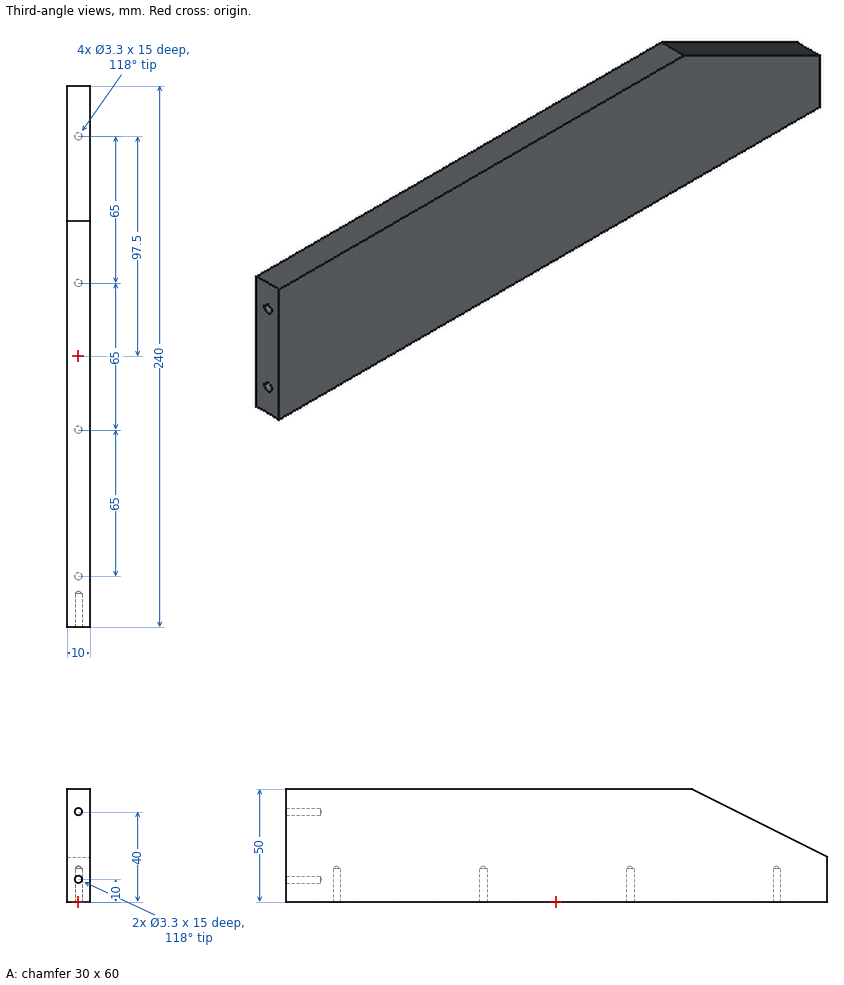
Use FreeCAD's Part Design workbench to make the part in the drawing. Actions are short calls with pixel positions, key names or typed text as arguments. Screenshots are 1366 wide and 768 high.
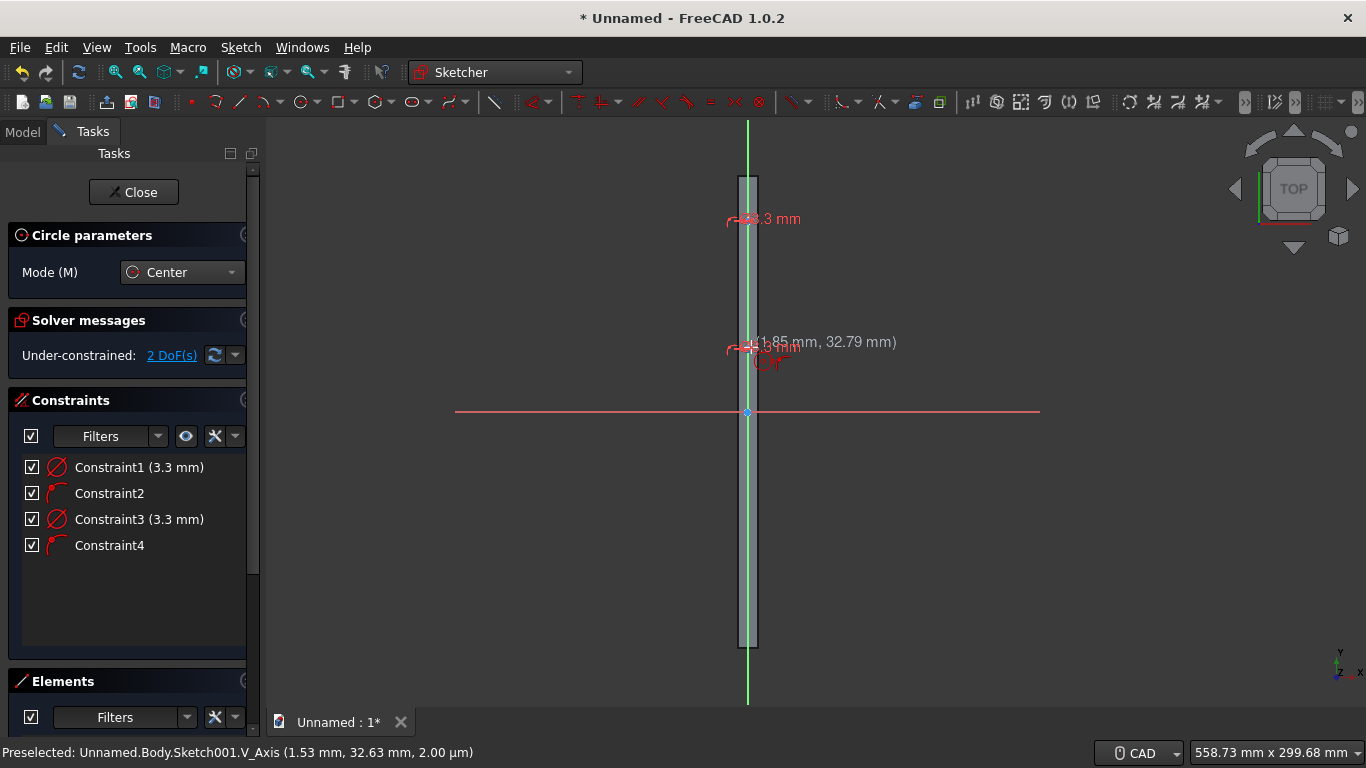
scroll(748, 476, up, 10)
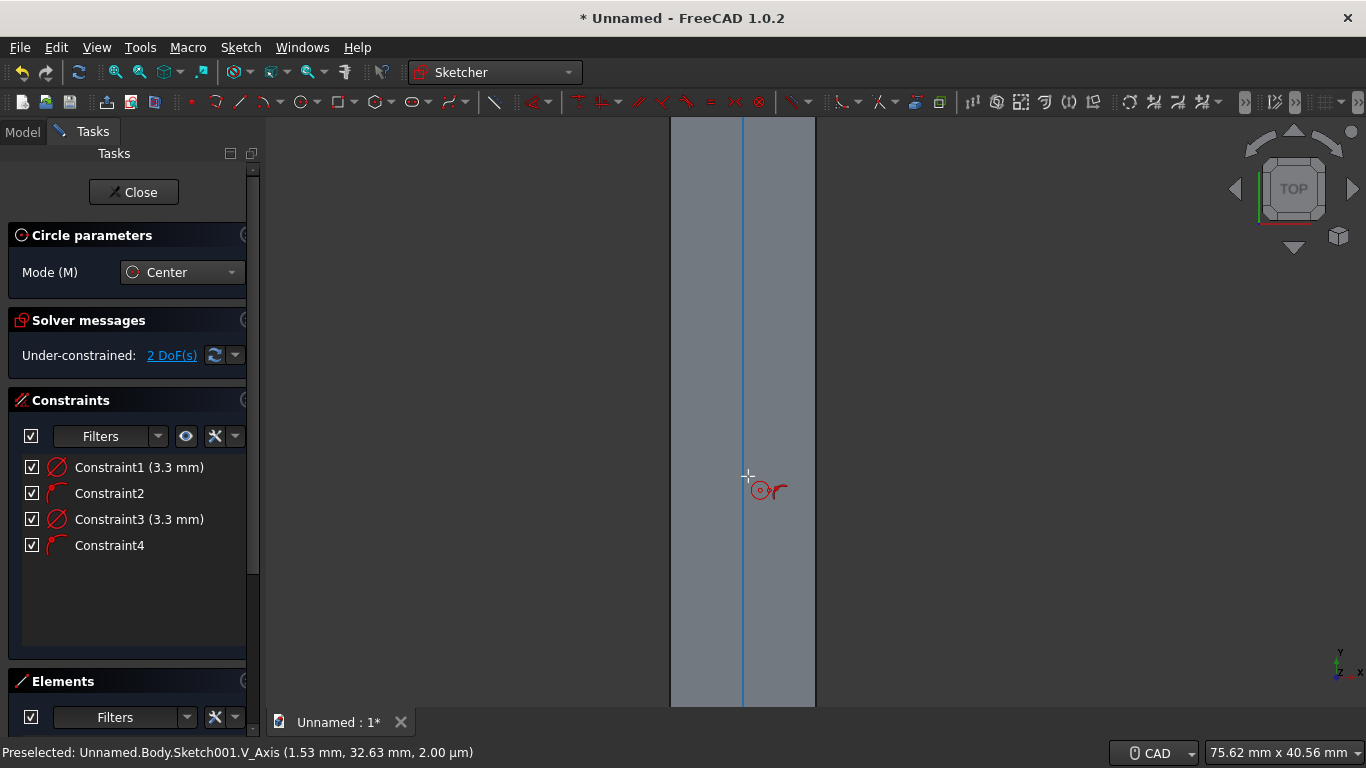
scroll(748, 477, down, 10)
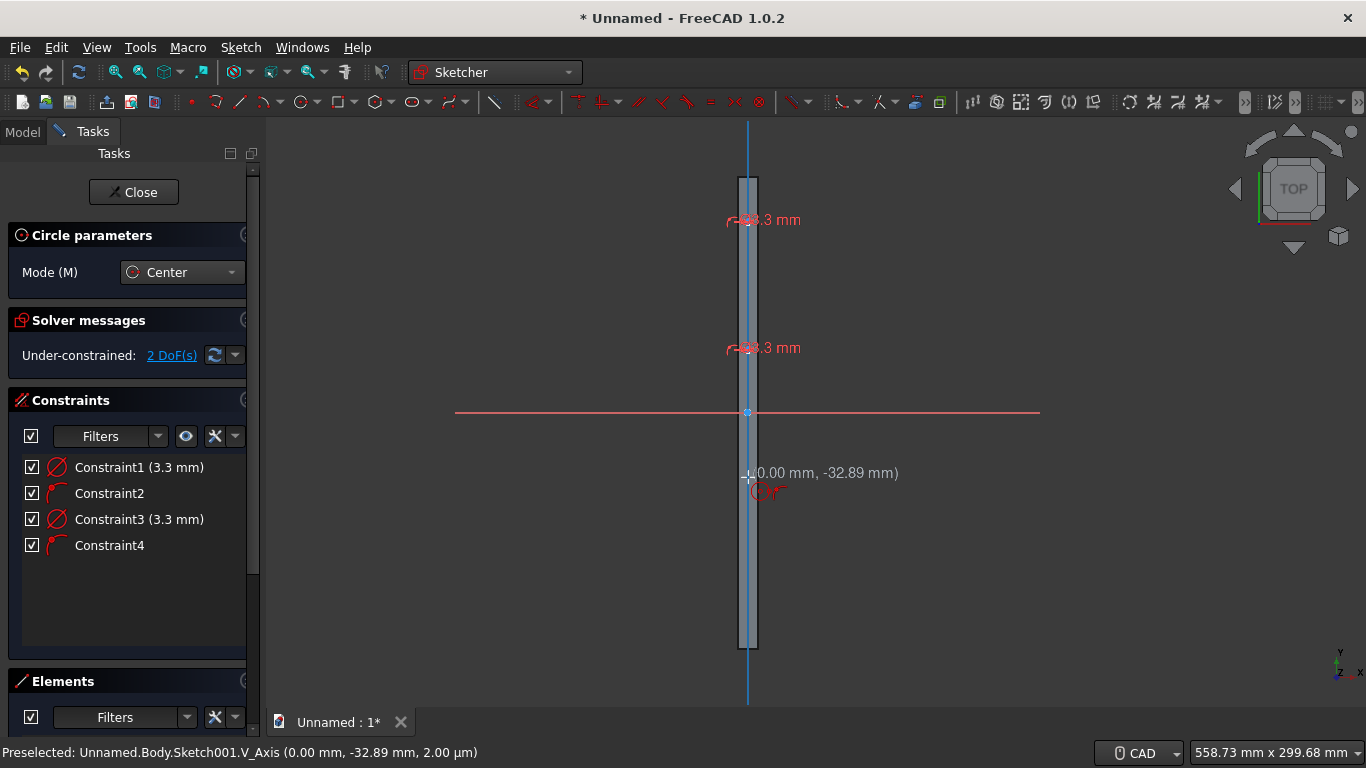
click(748, 477)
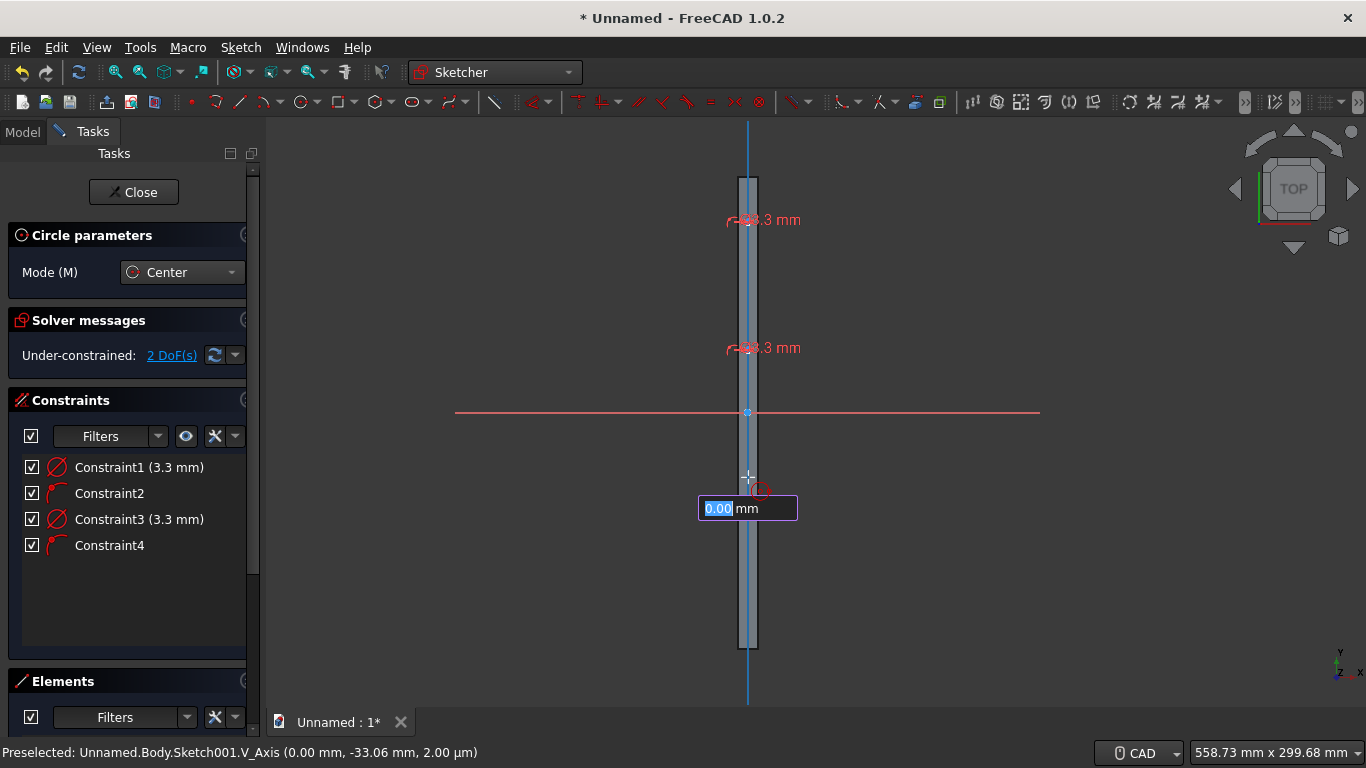
scroll(751, 476, up, 9)
move(747, 472)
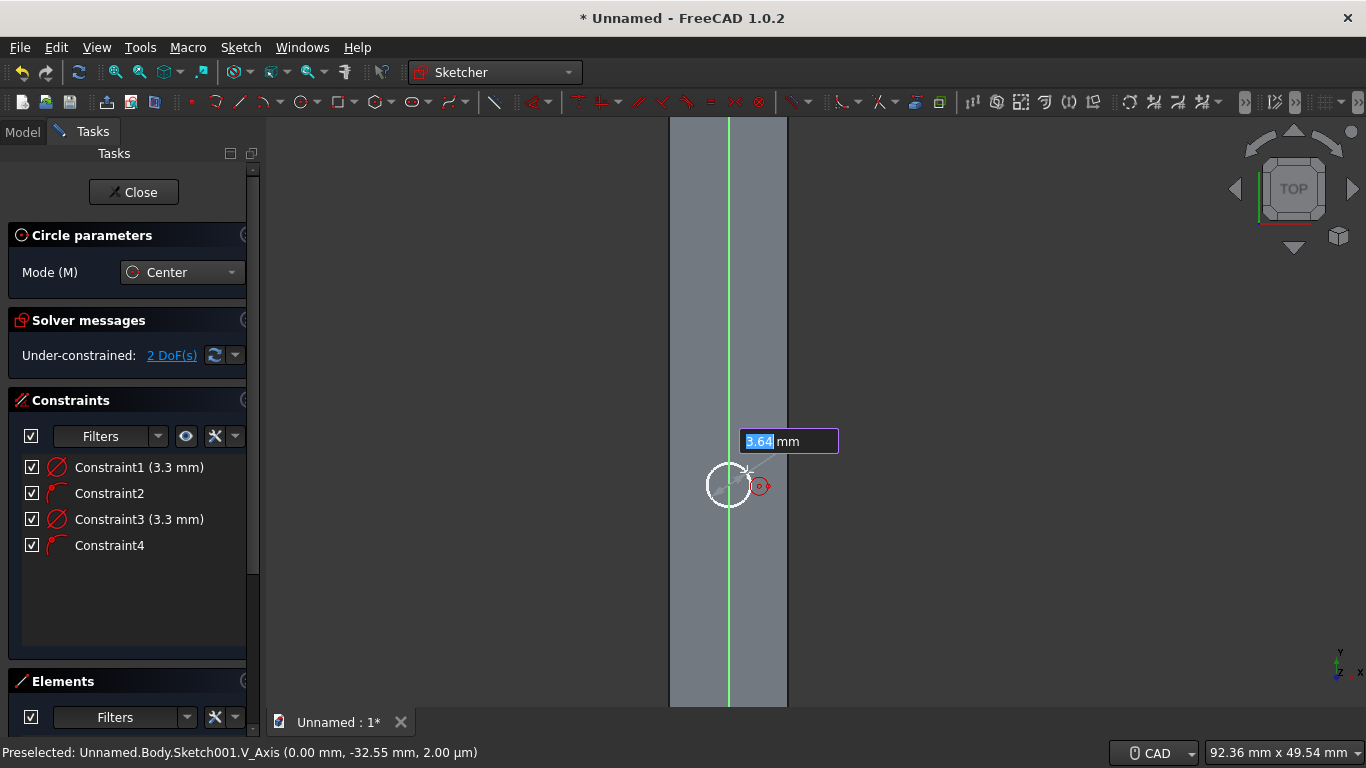
text(3.3)
key(Return)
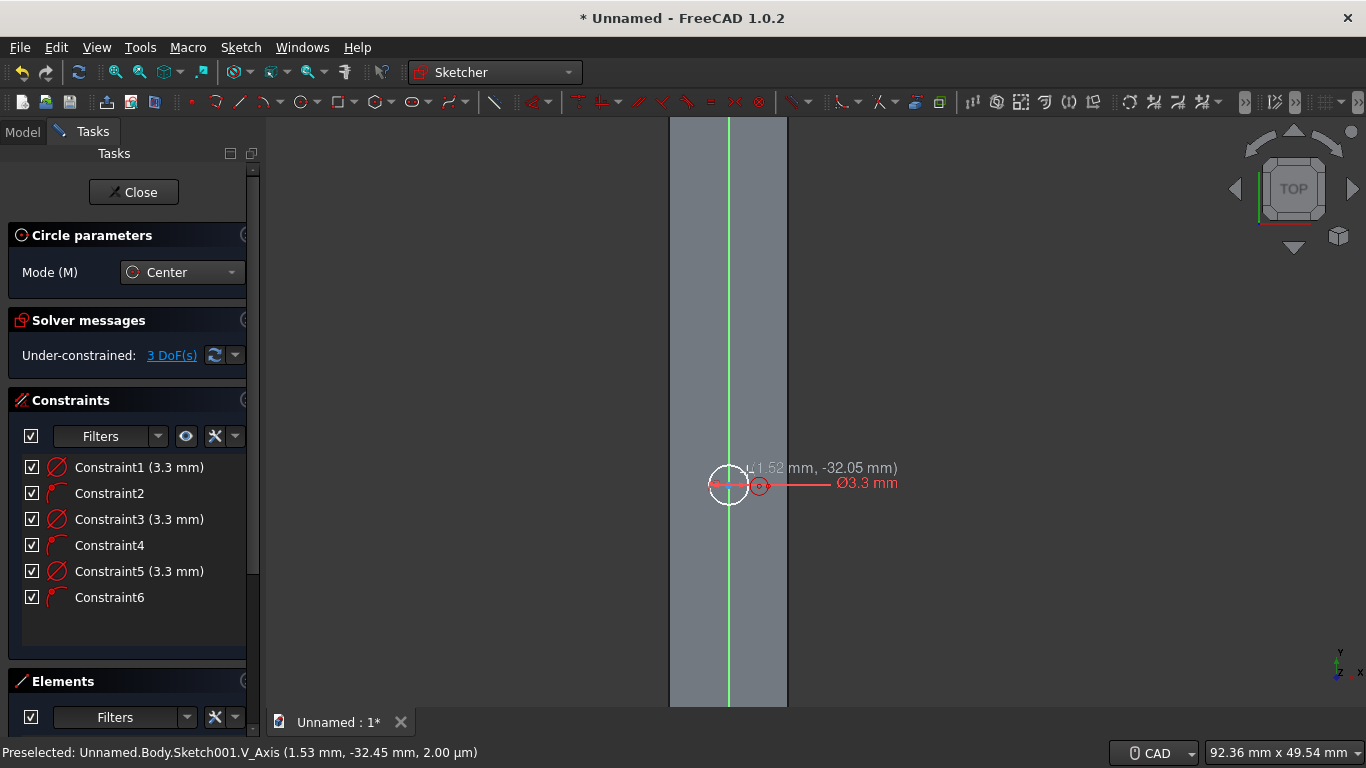
scroll(751, 476, down, 9)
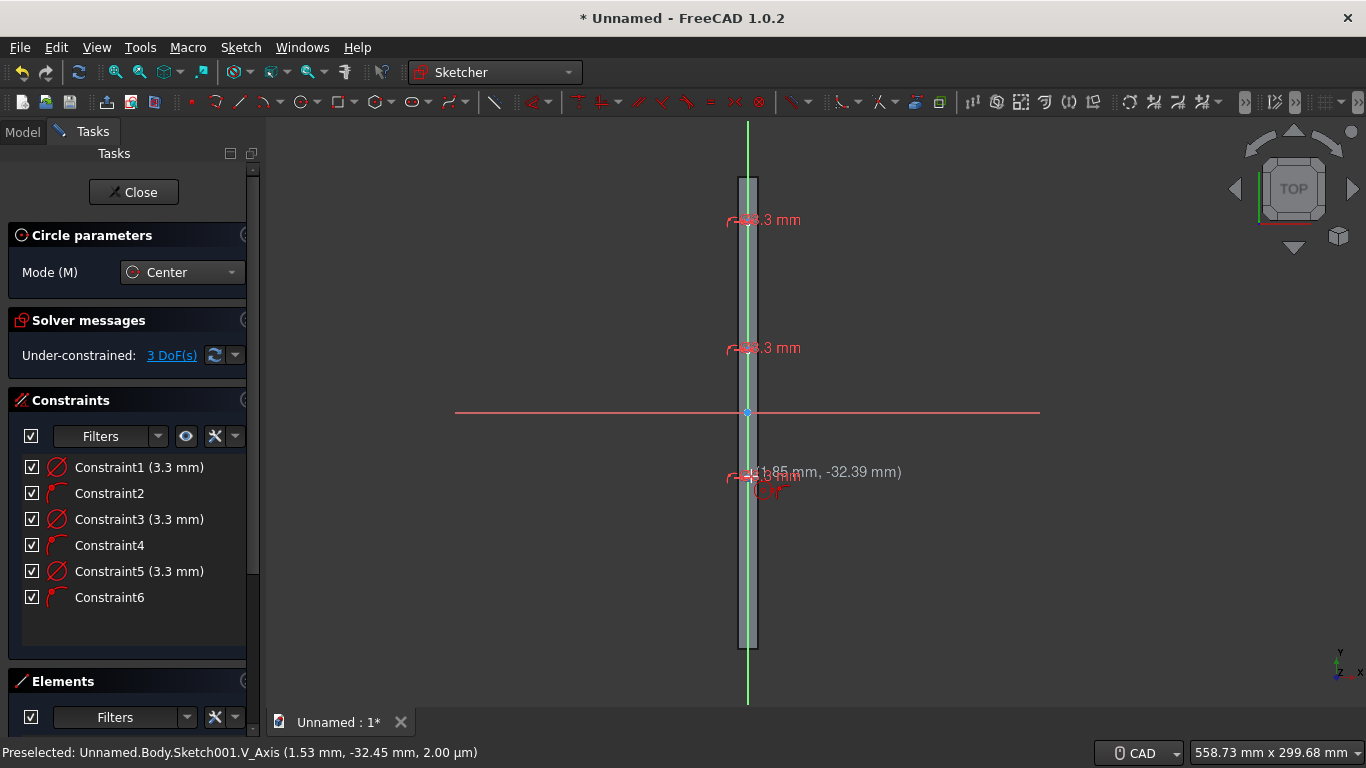
scroll(748, 605, up, 10)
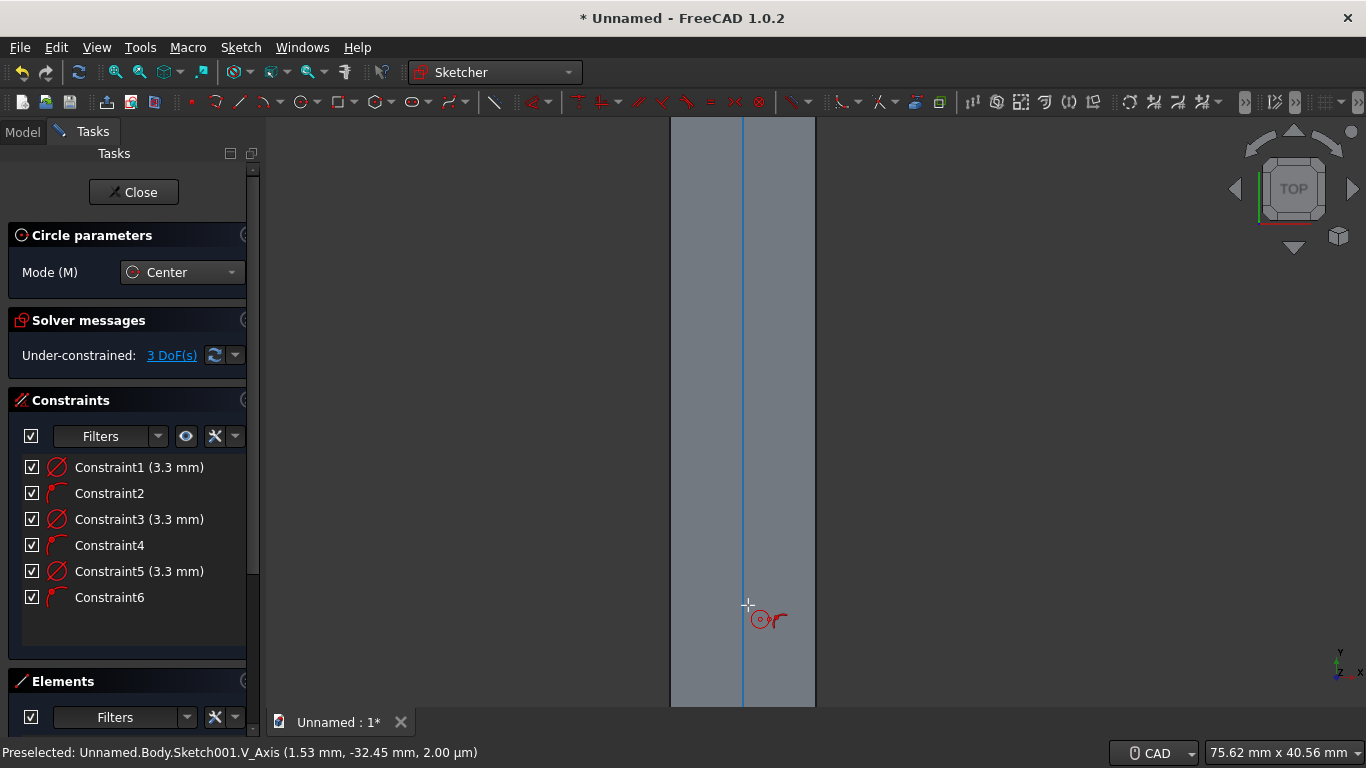
scroll(748, 605, down, 10)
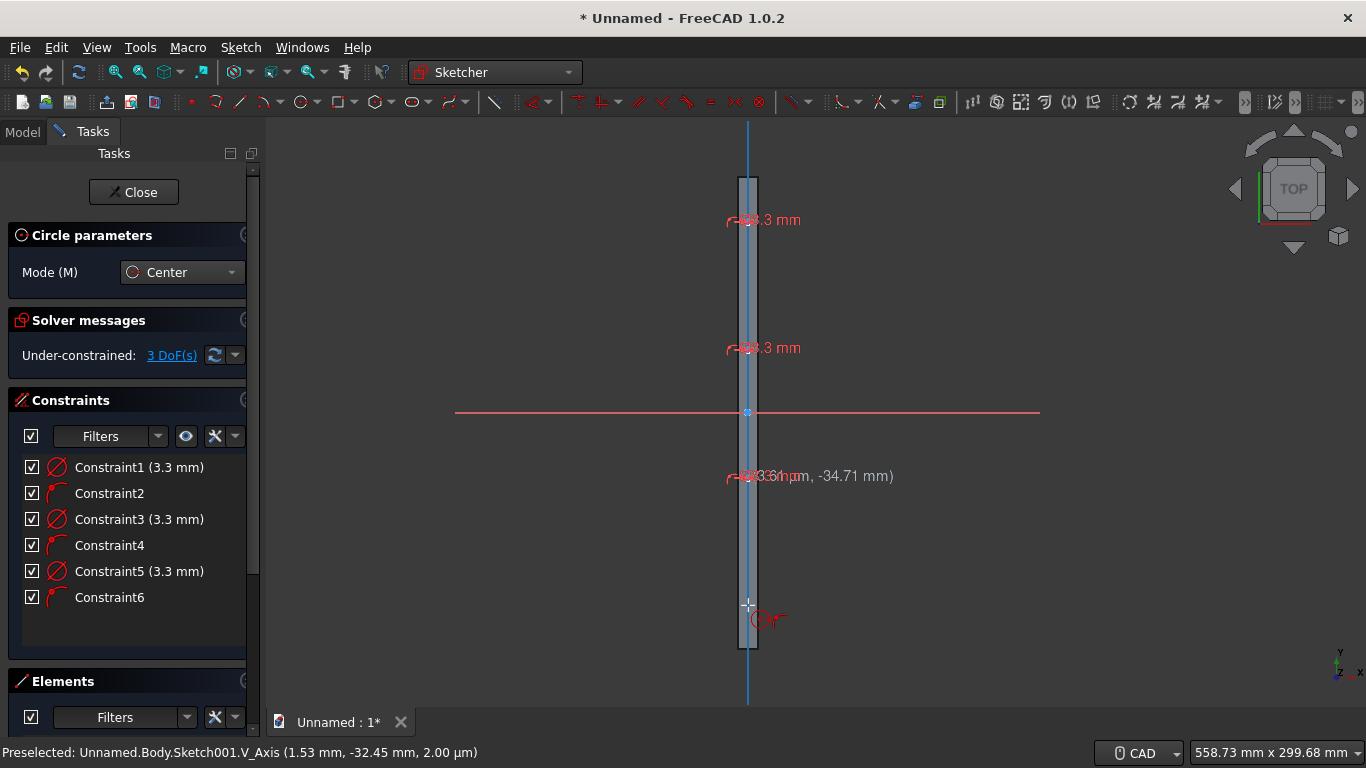
click(748, 605)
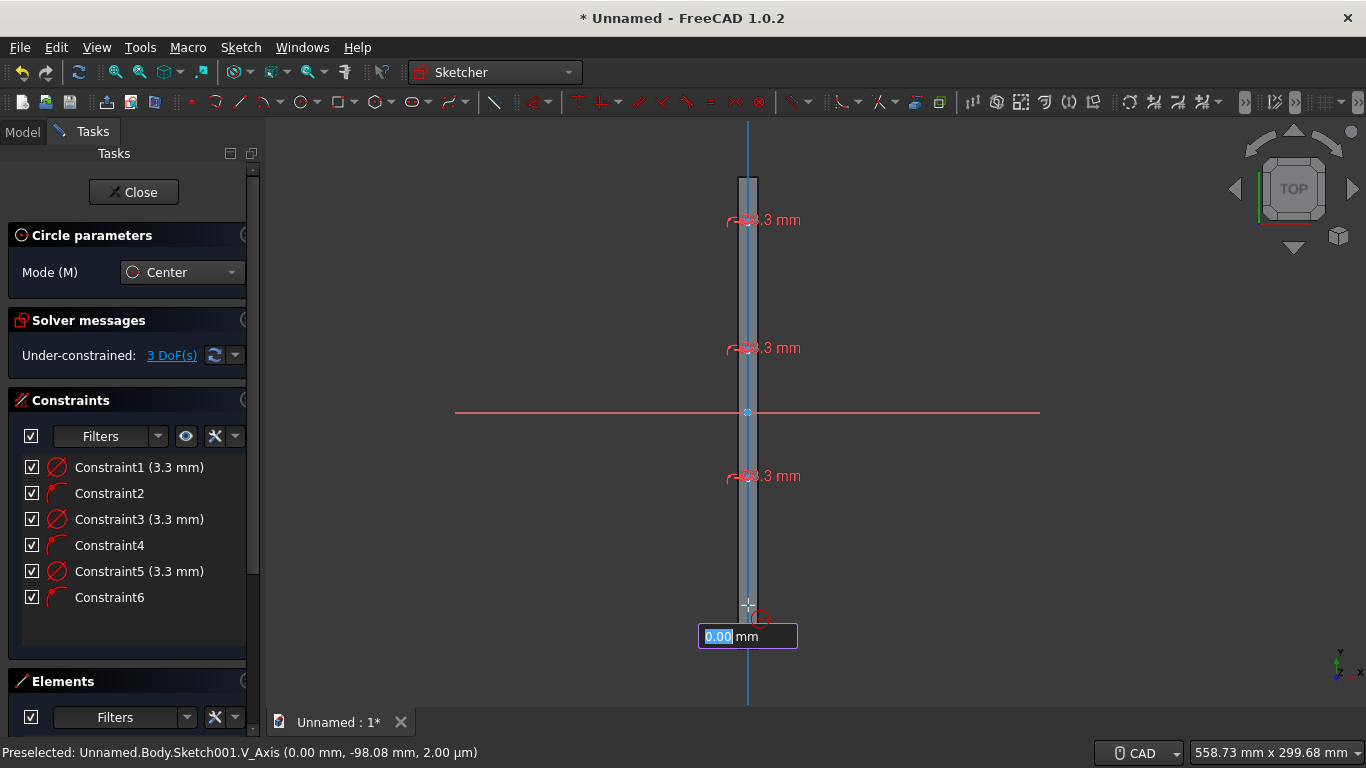
scroll(751, 604, up, 9)
move(747, 598)